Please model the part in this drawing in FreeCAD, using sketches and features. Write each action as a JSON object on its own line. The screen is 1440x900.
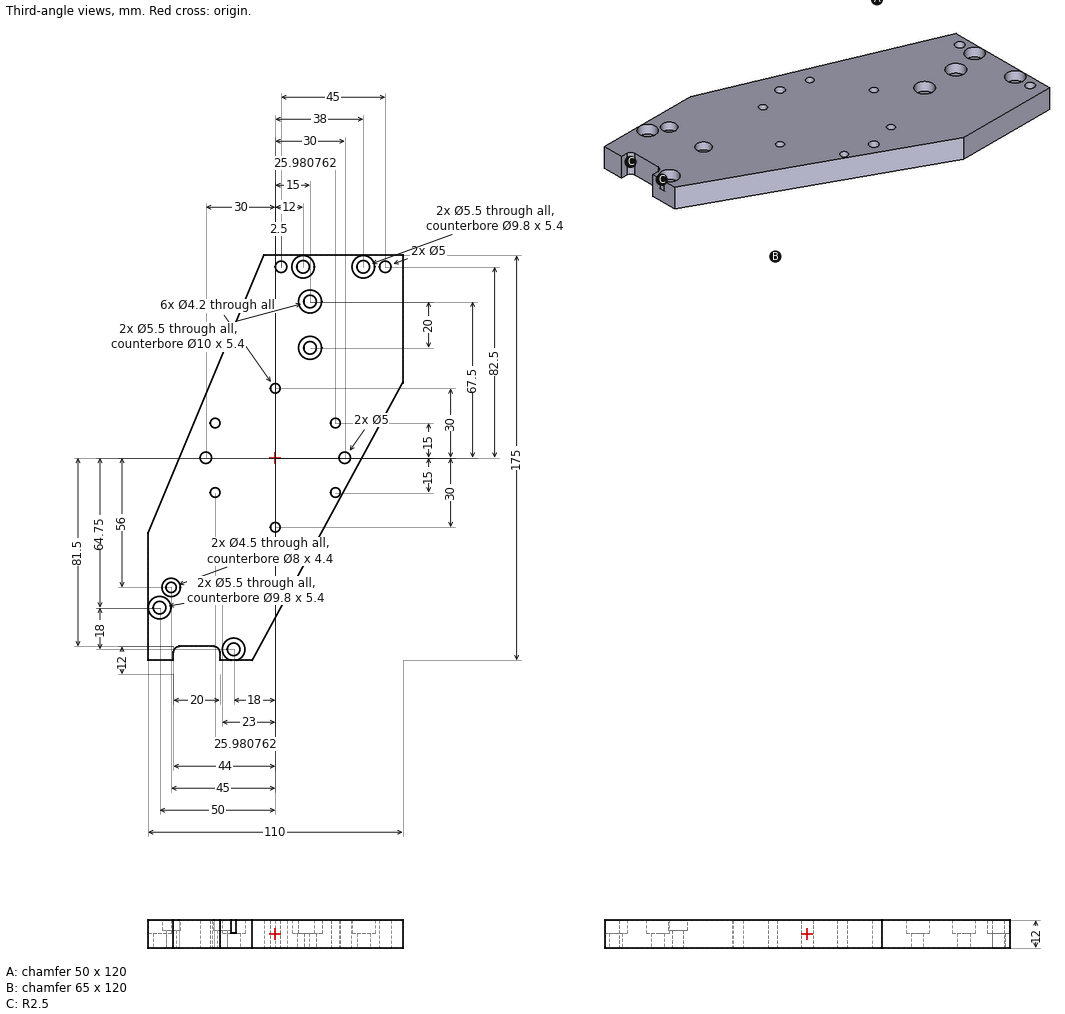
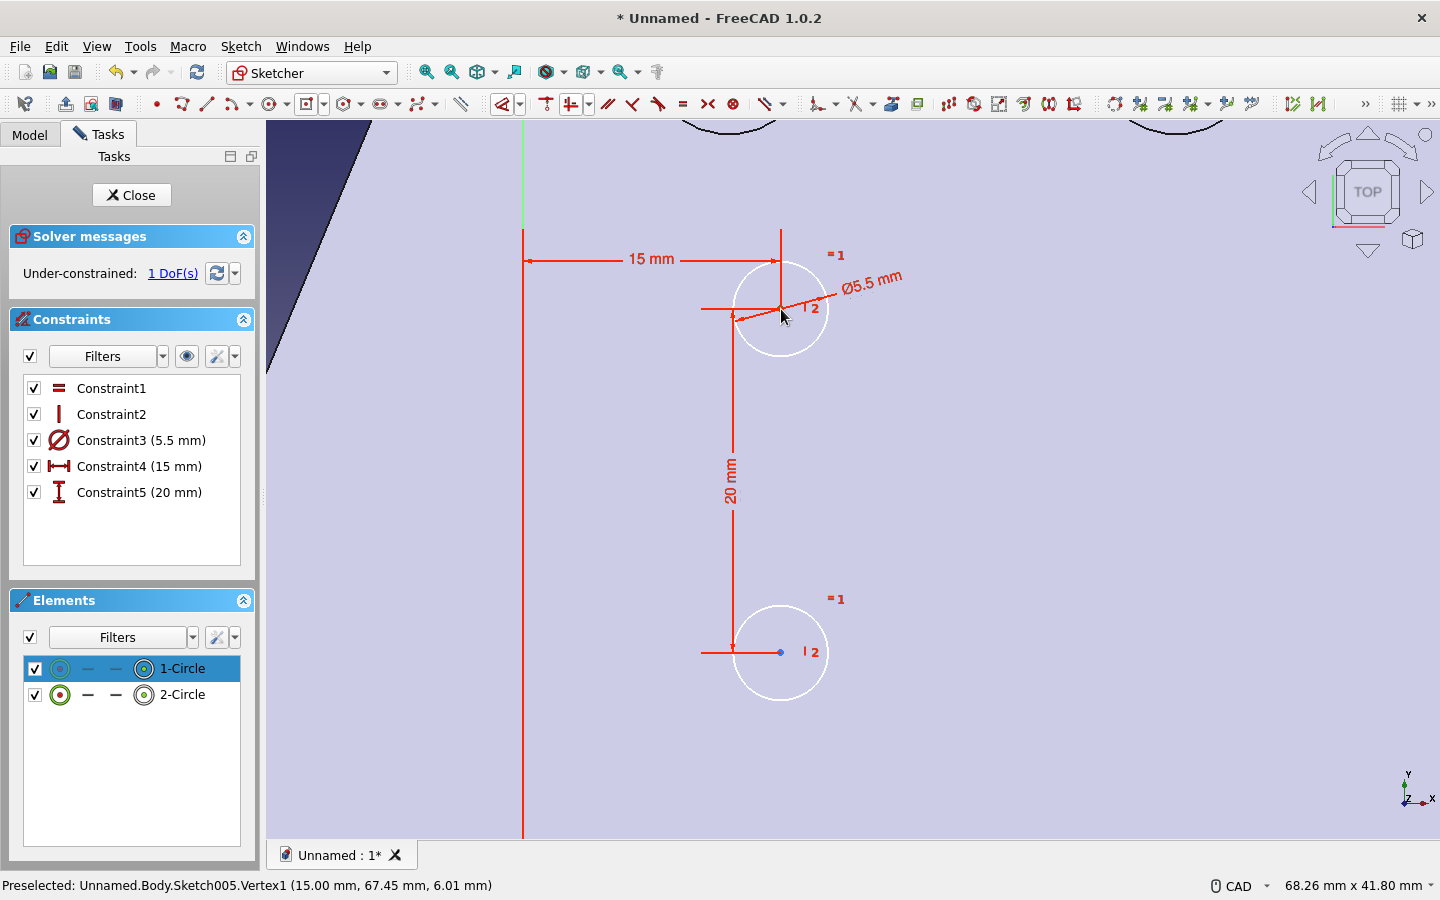
{"action": "key", "text": "i"}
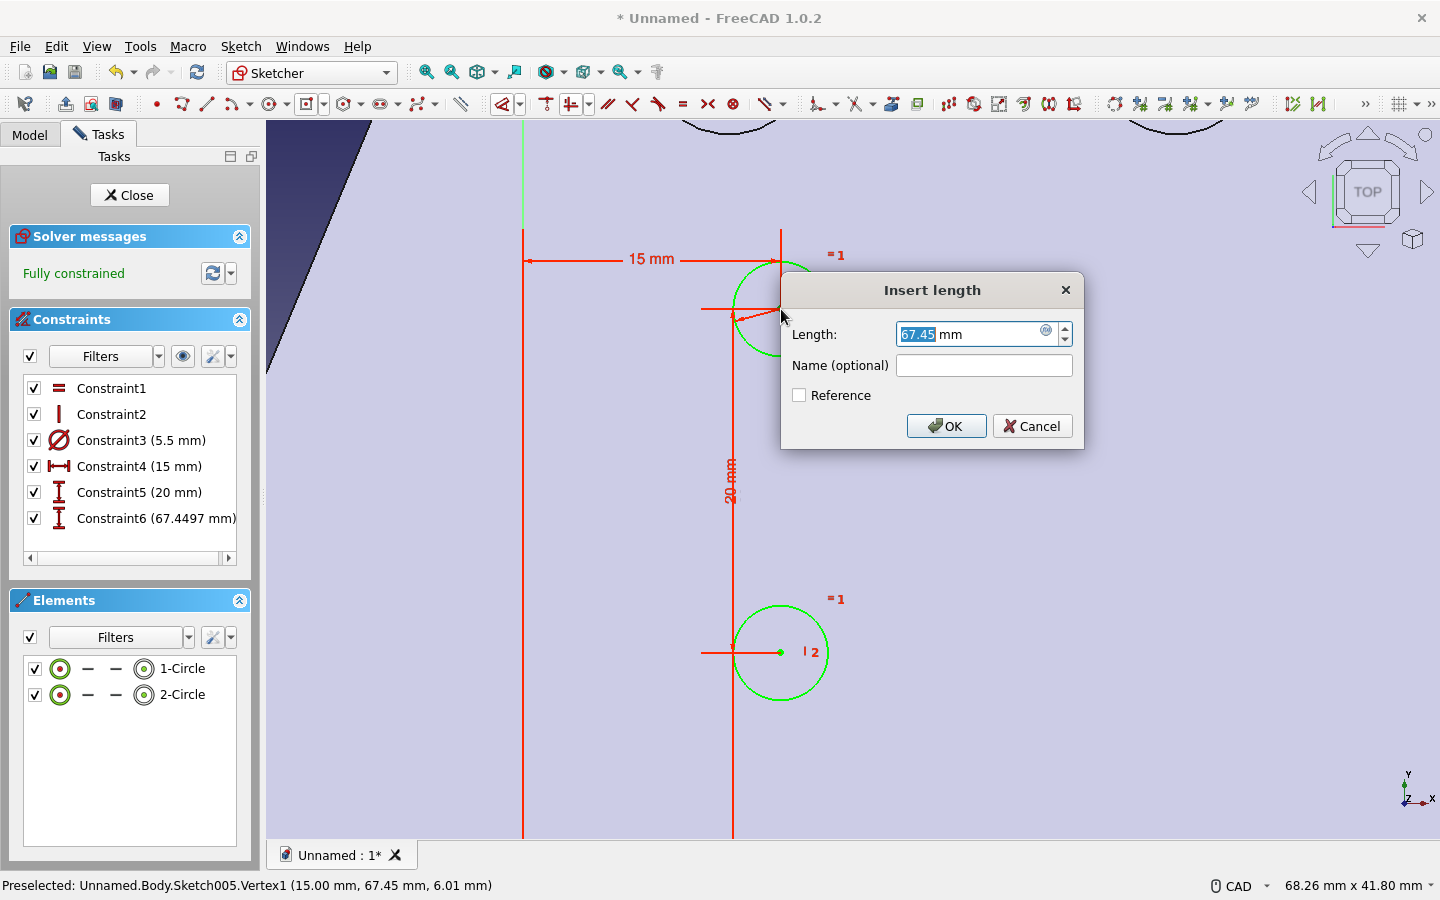
{"action": "type", "text": "67.5"}
{"action": "key", "text": "Return"}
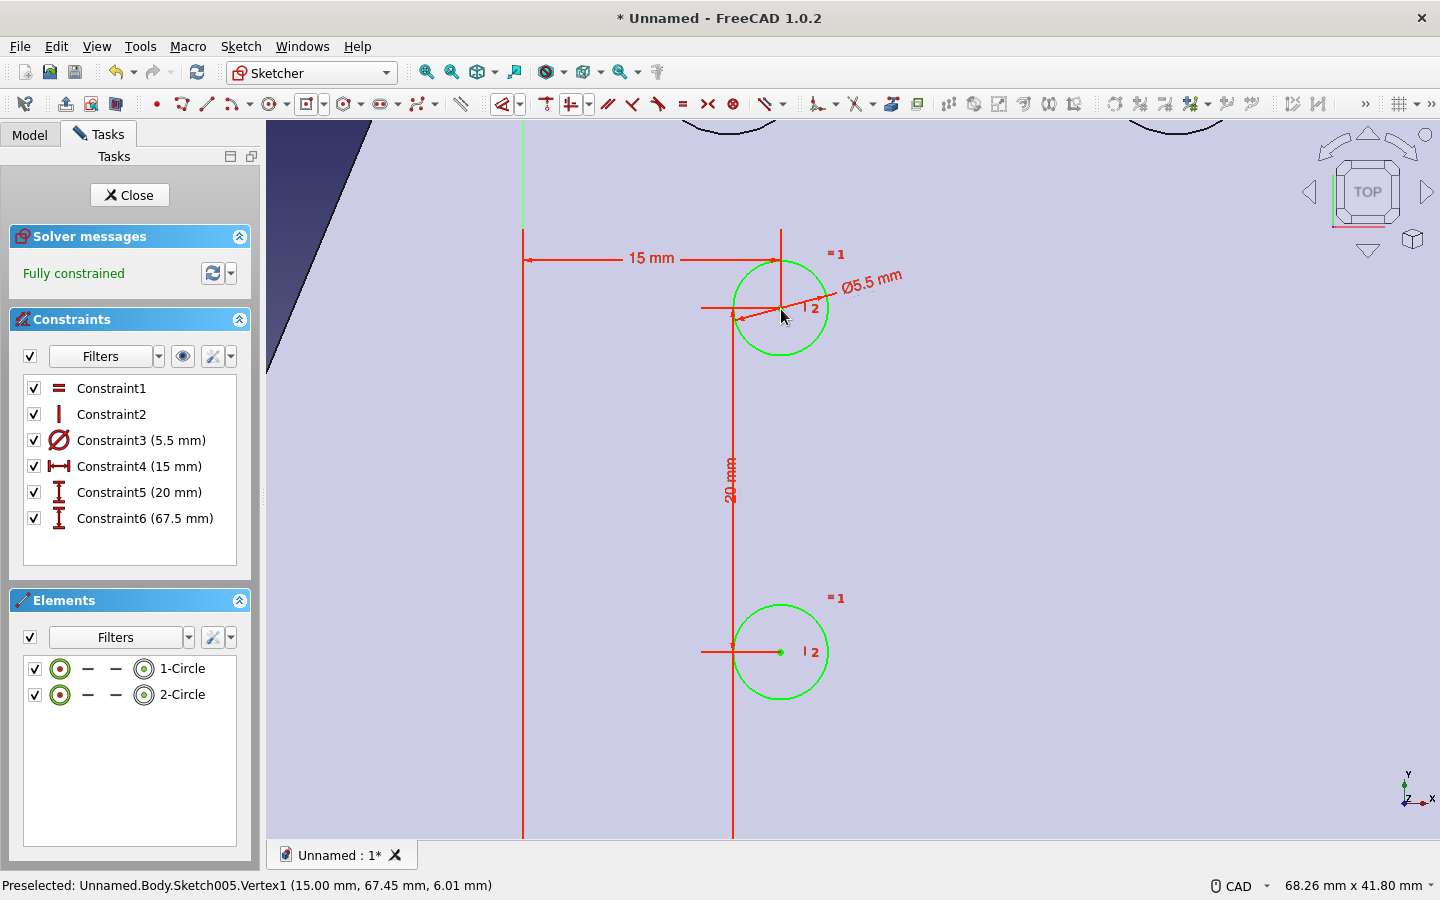
{"action": "left_click", "coordinate": [130, 195]}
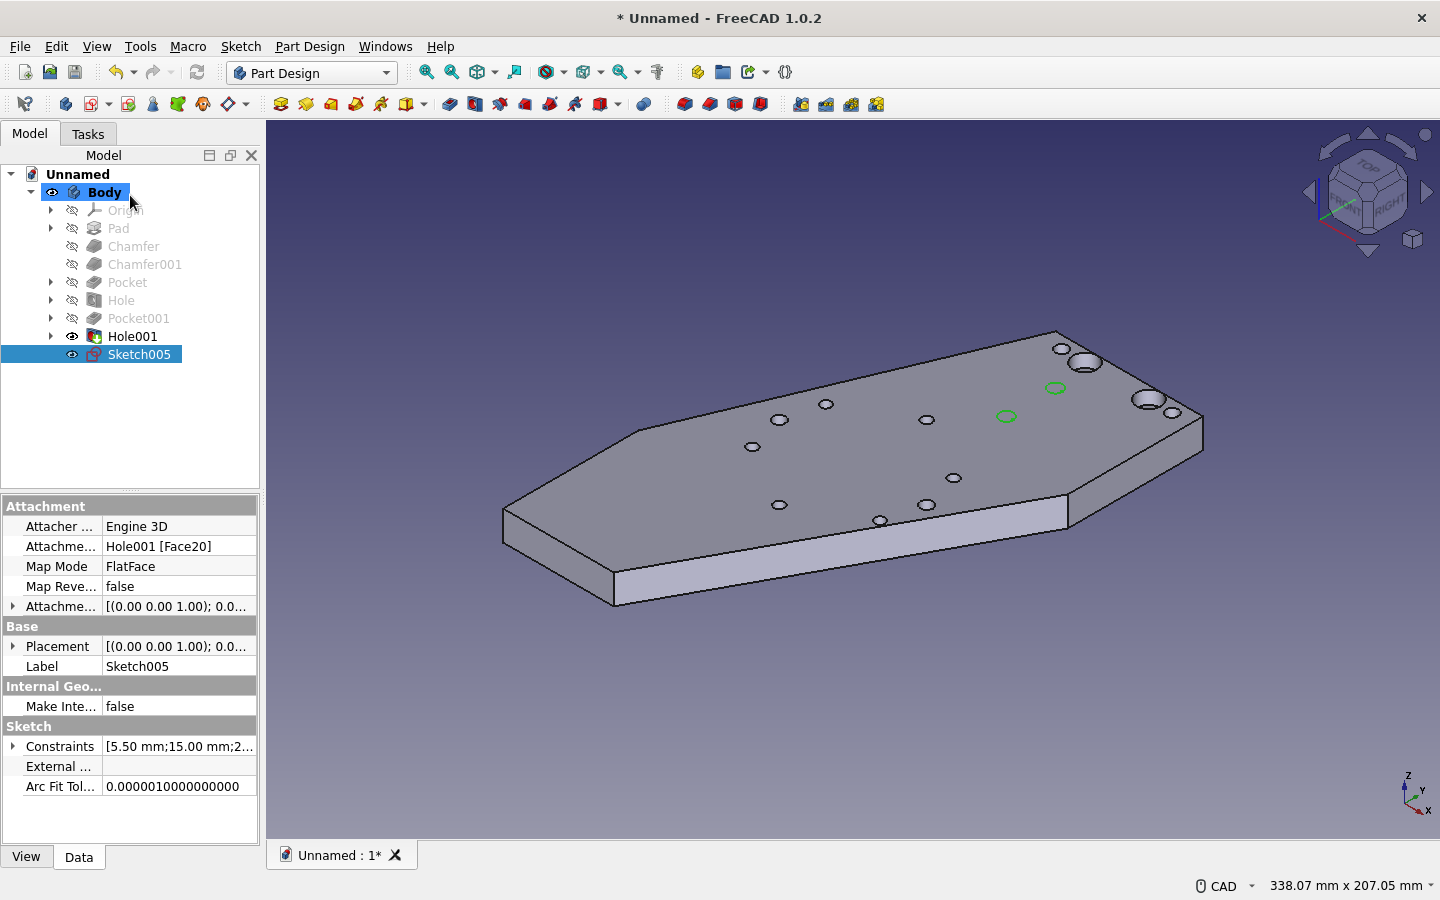
{"action": "left_click", "coordinate": [475, 104]}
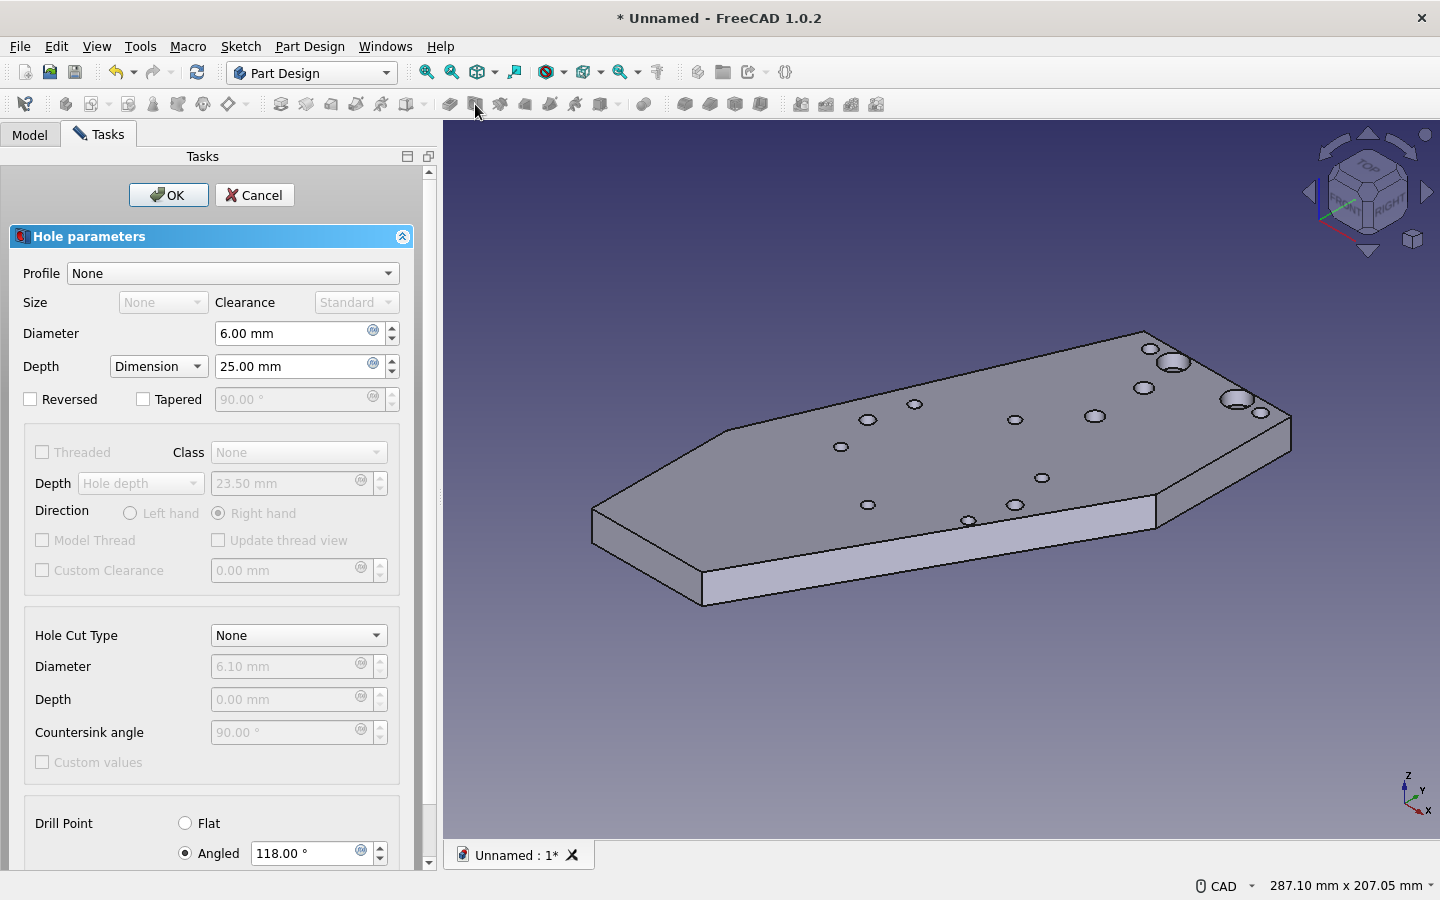
{"action": "triple_click", "coordinate": [300, 334]}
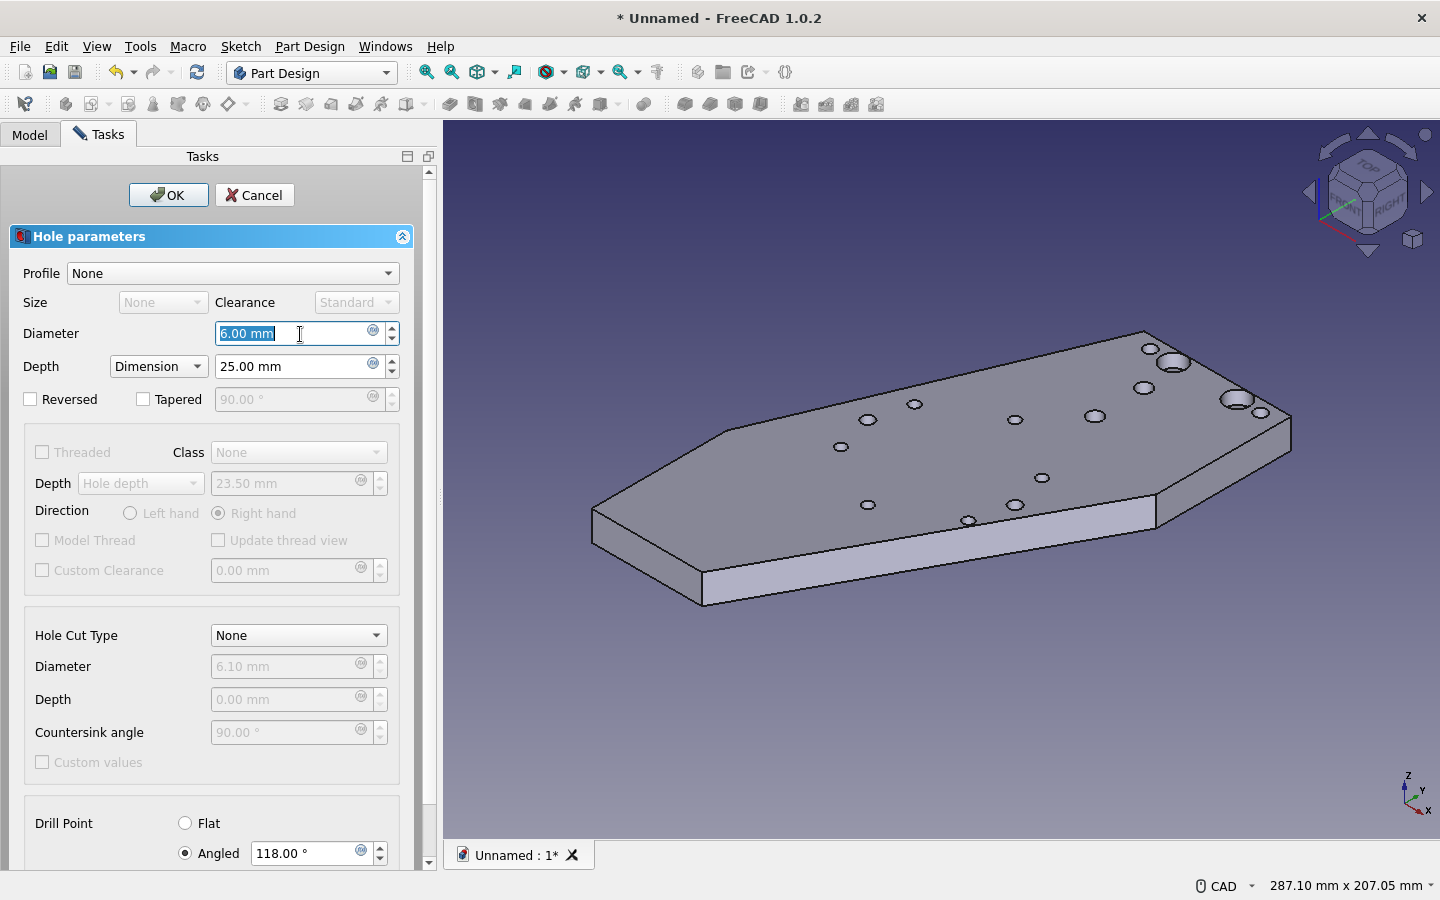
{"action": "type", "text": "5.5"}
{"action": "key", "text": "Tab"}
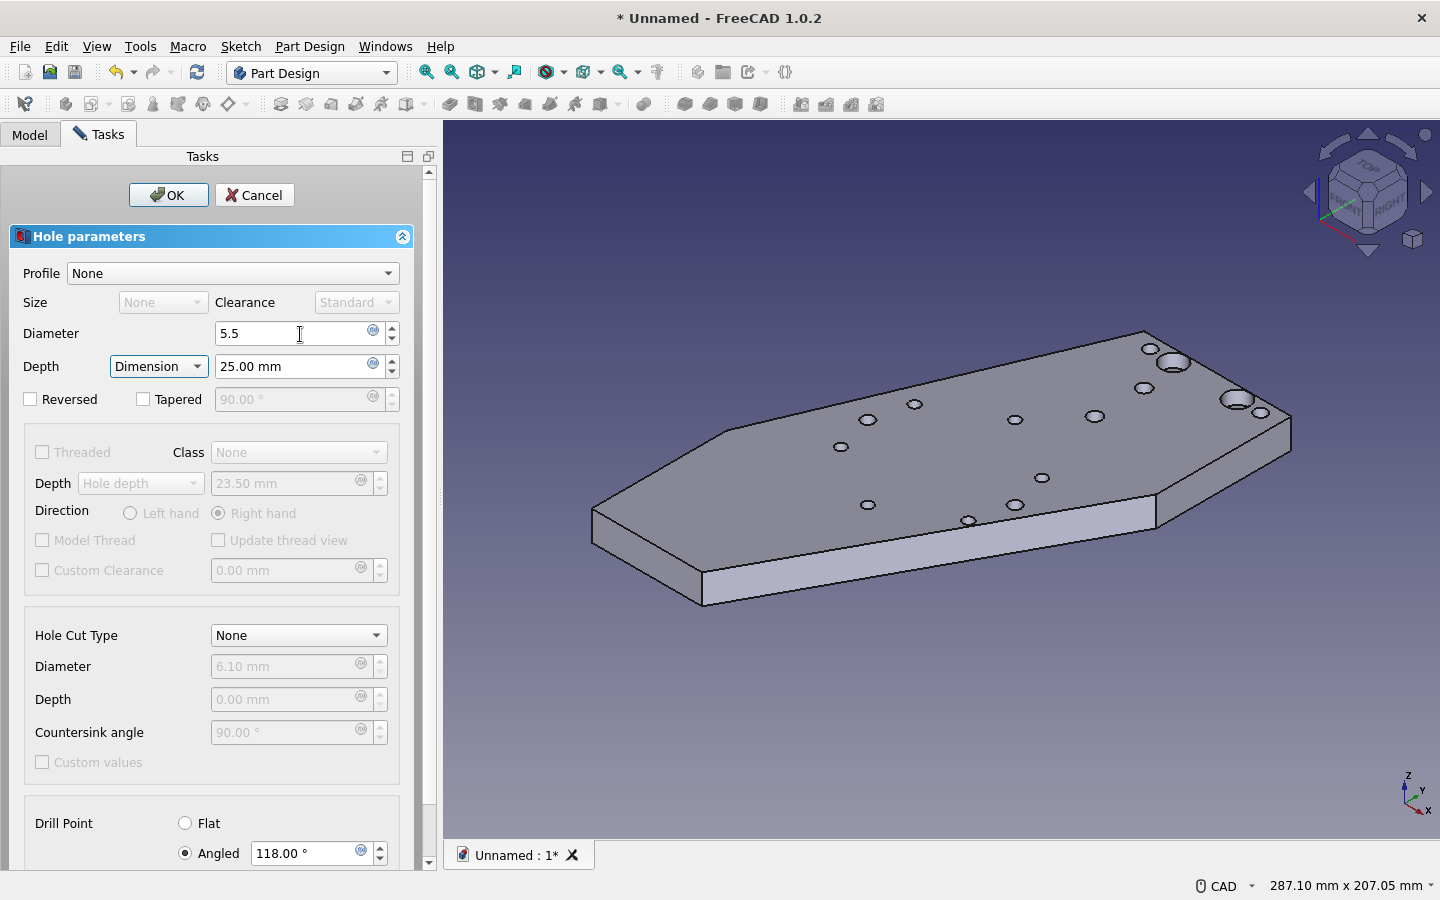
{"action": "left_click", "coordinate": [160, 366]}